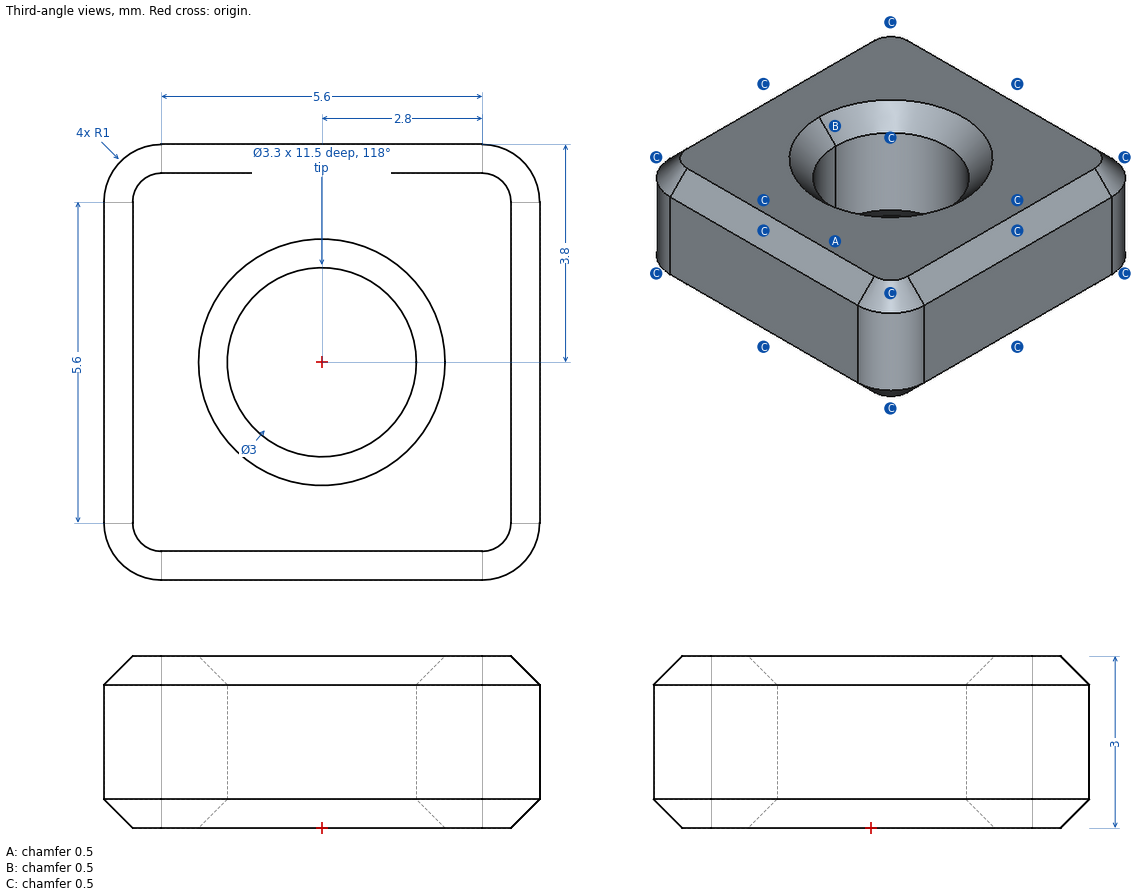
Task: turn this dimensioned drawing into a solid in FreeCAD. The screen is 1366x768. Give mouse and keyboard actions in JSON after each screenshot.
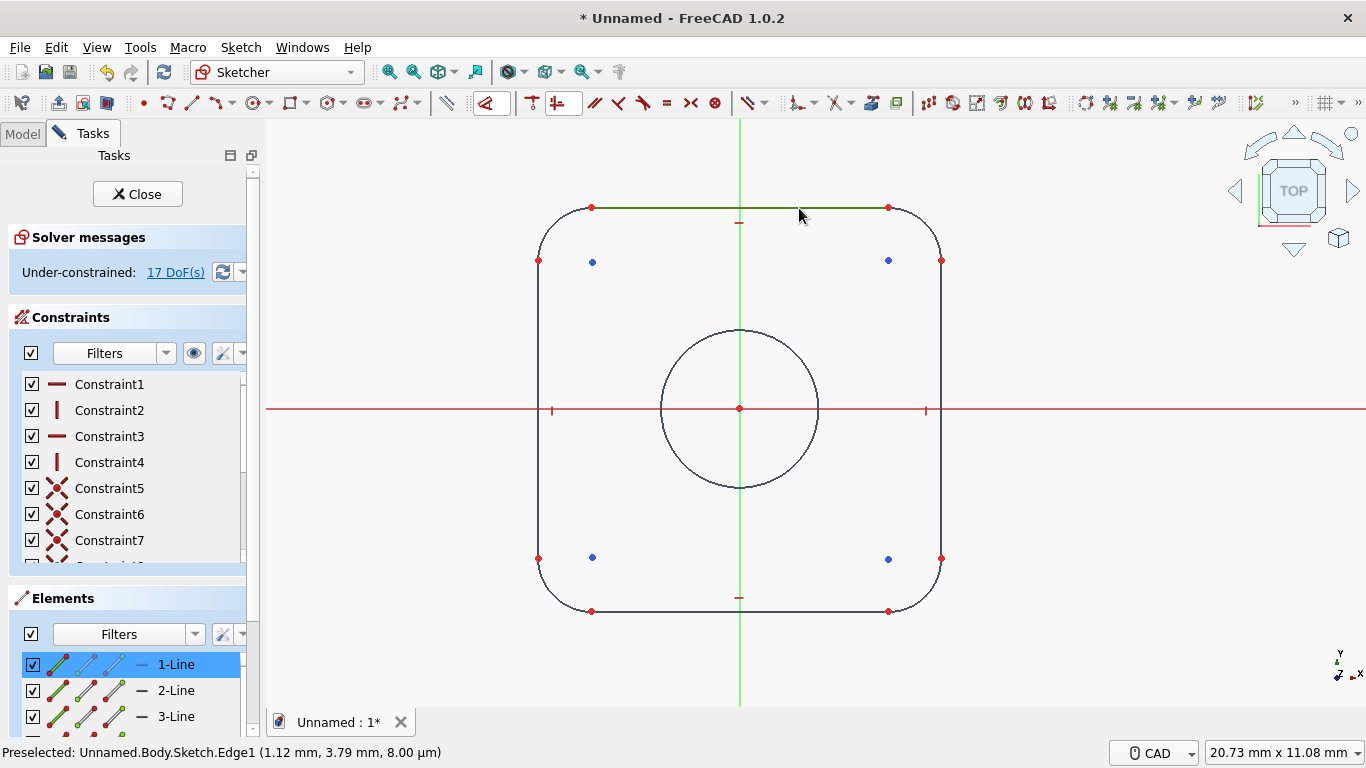
{"action": "left_click", "coordinate": [567, 214]}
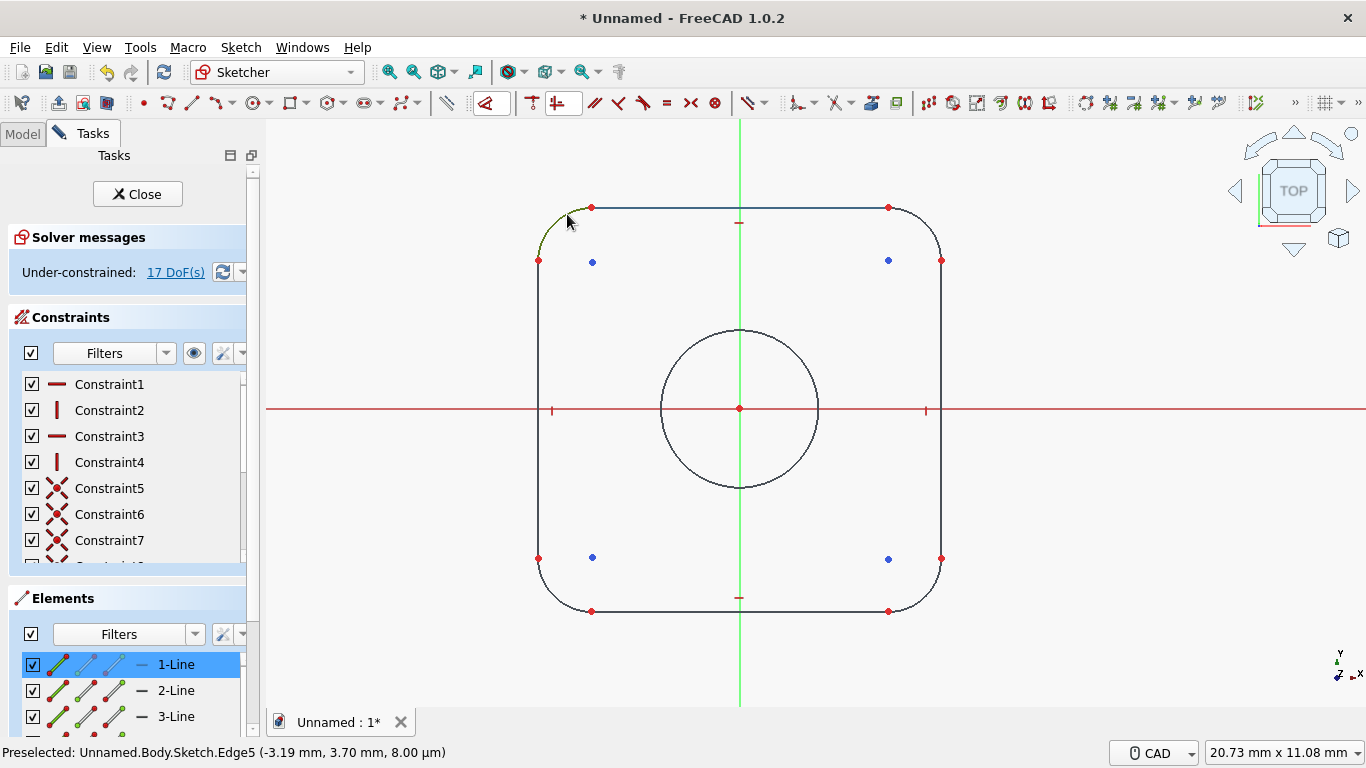
{"action": "key", "text": "t"}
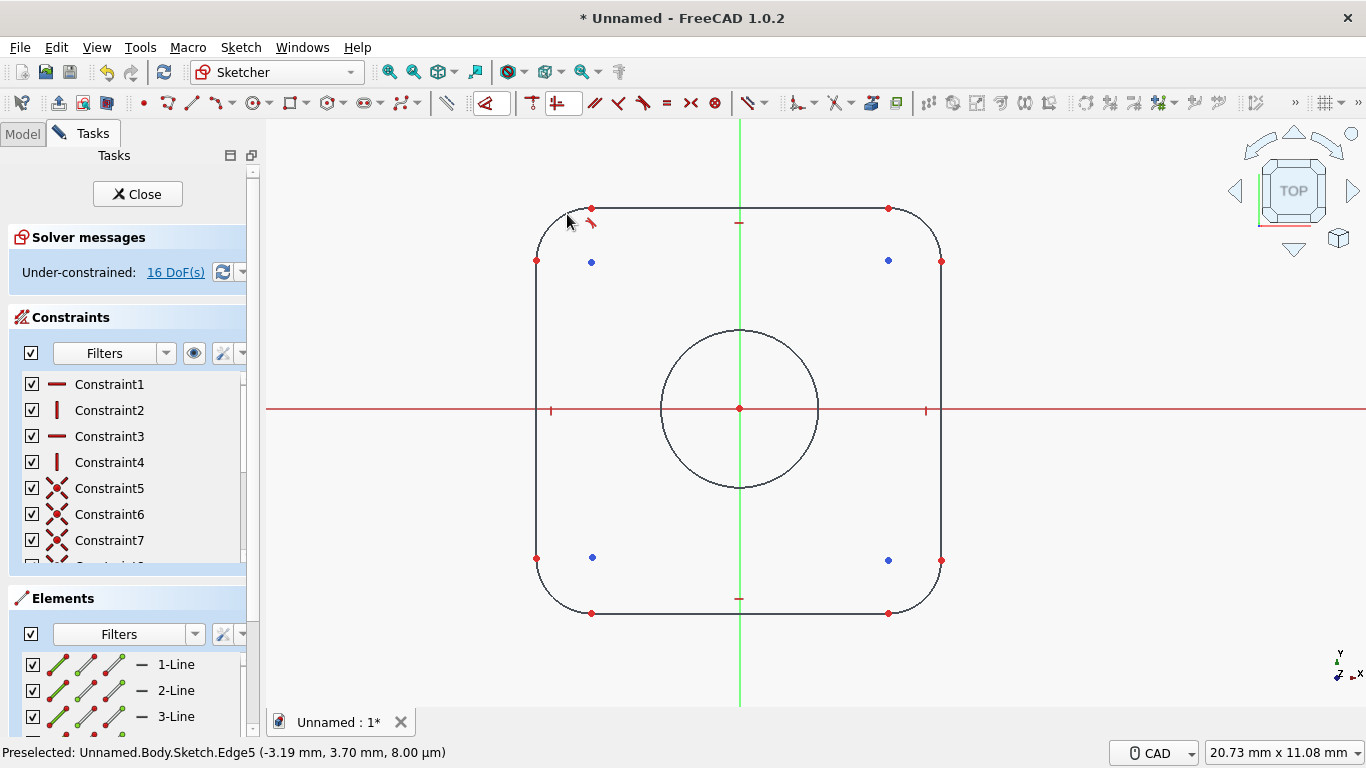
{"action": "left_click", "coordinate": [799, 208]}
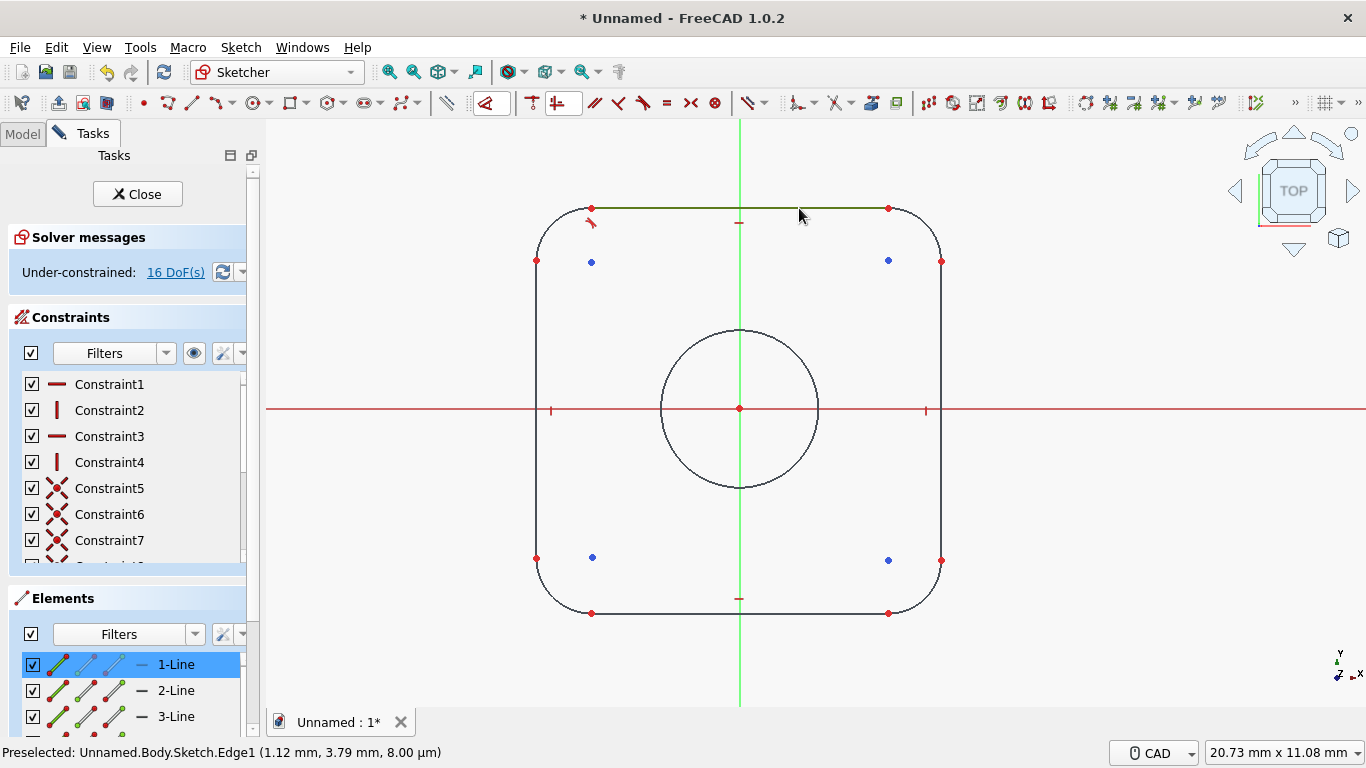
{"action": "left_click", "coordinate": [935, 237]}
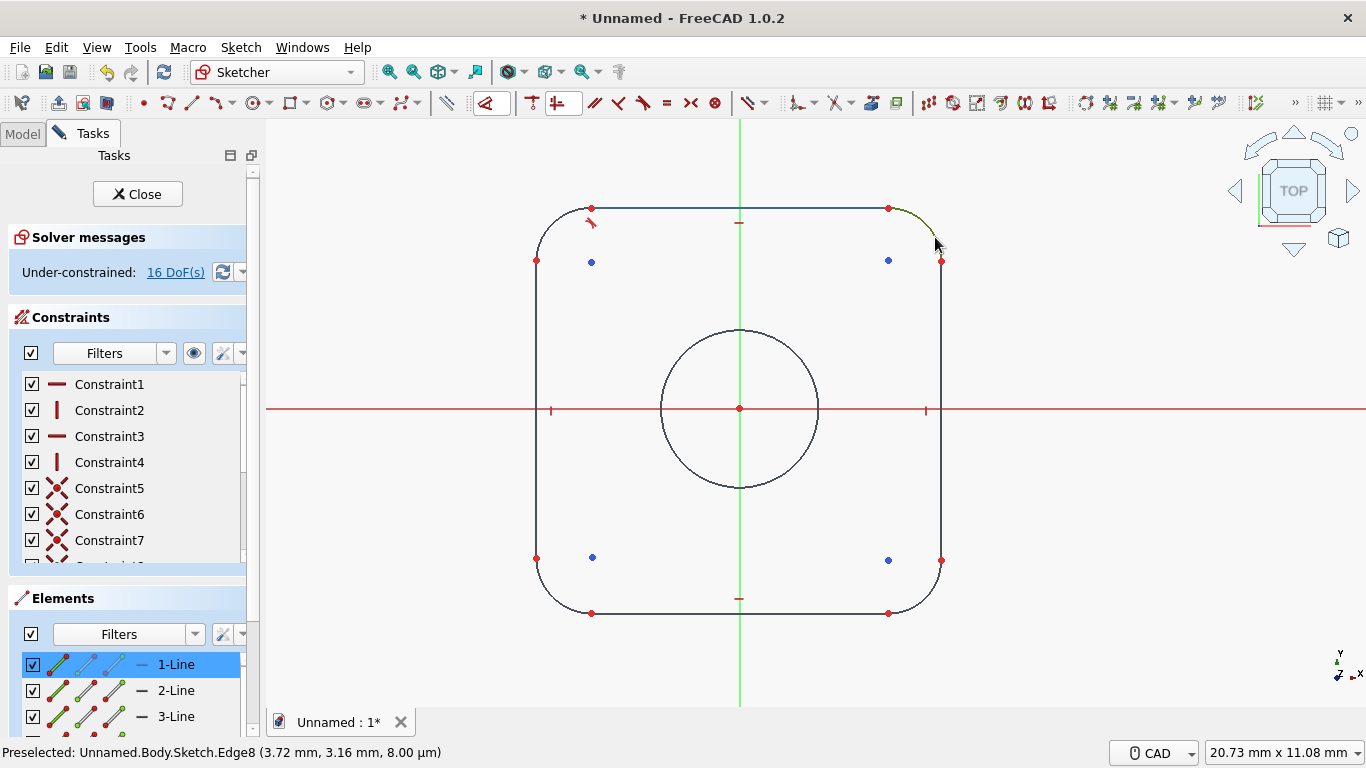
{"action": "left_click", "coordinate": [644, 104]}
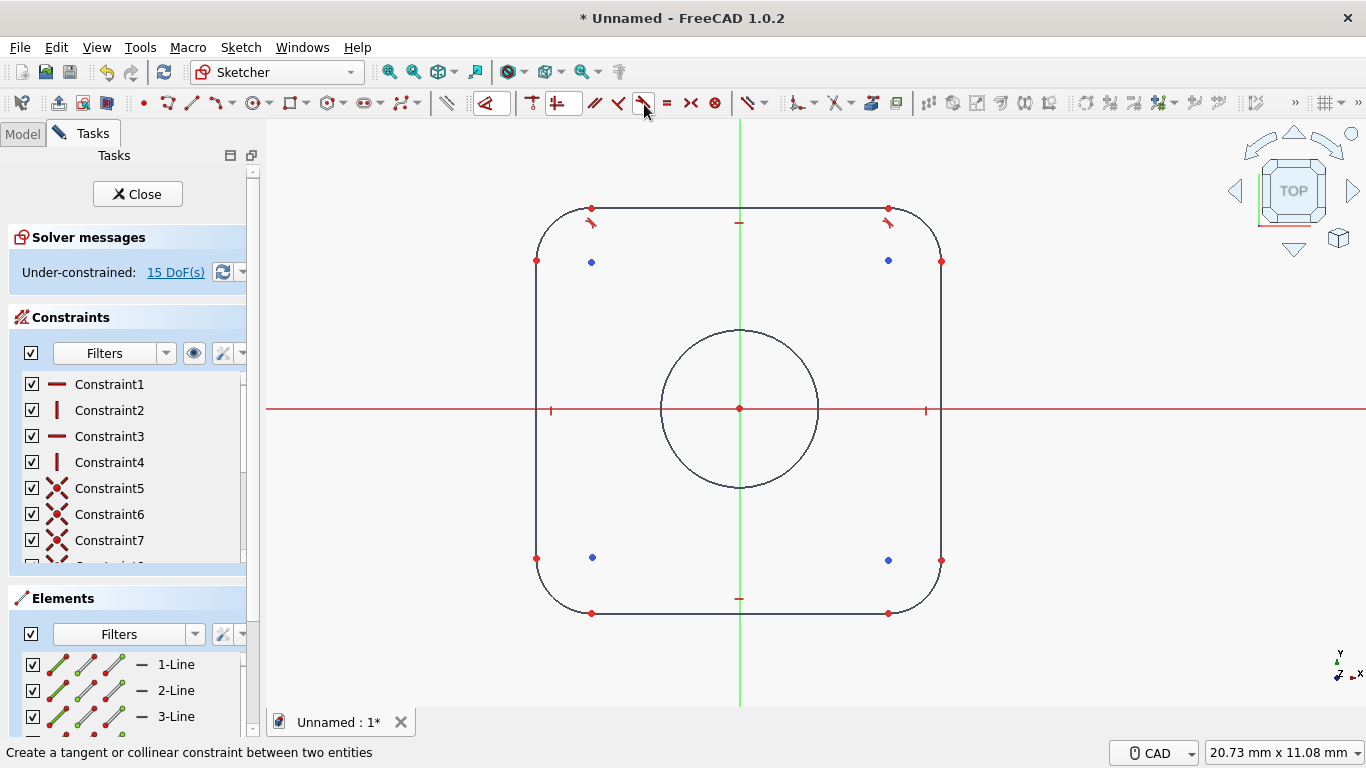
{"action": "left_click", "coordinate": [536, 350]}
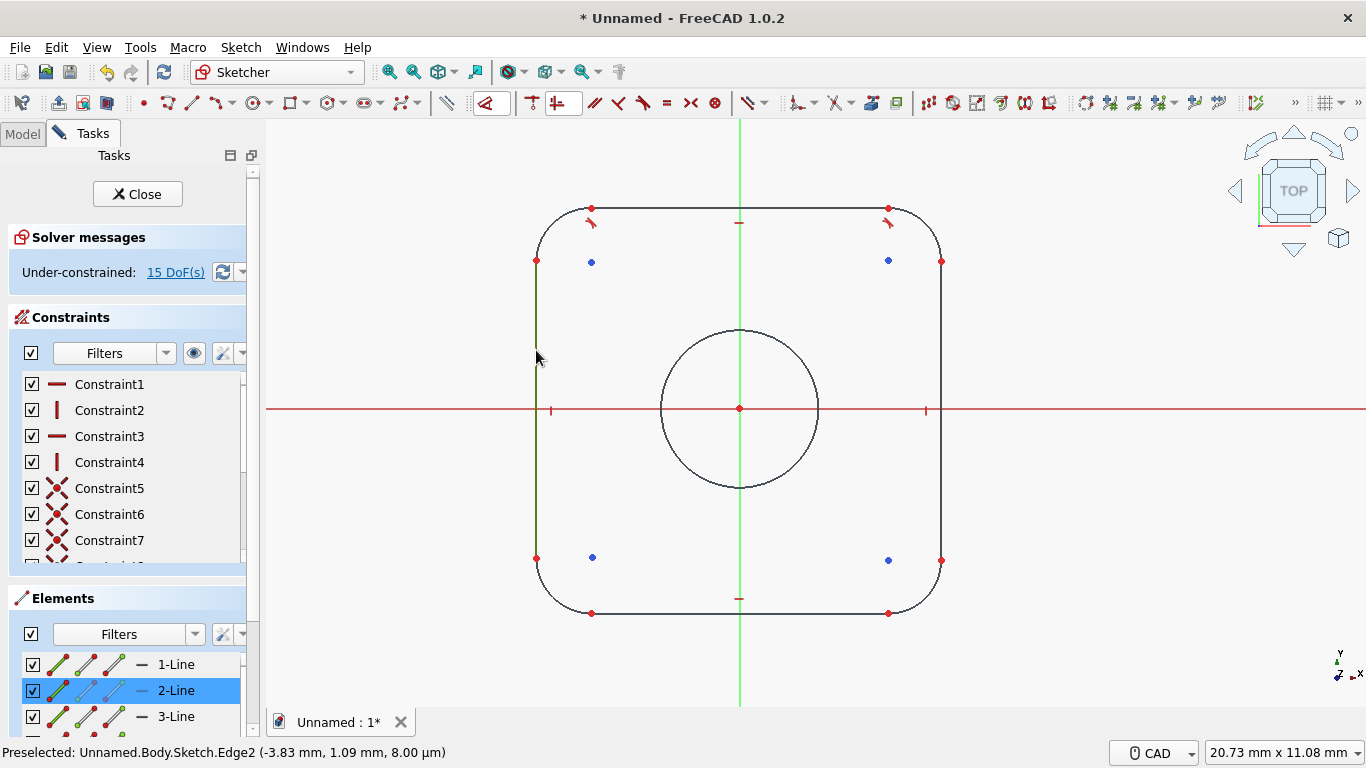
{"action": "left_click", "coordinate": [567, 214]}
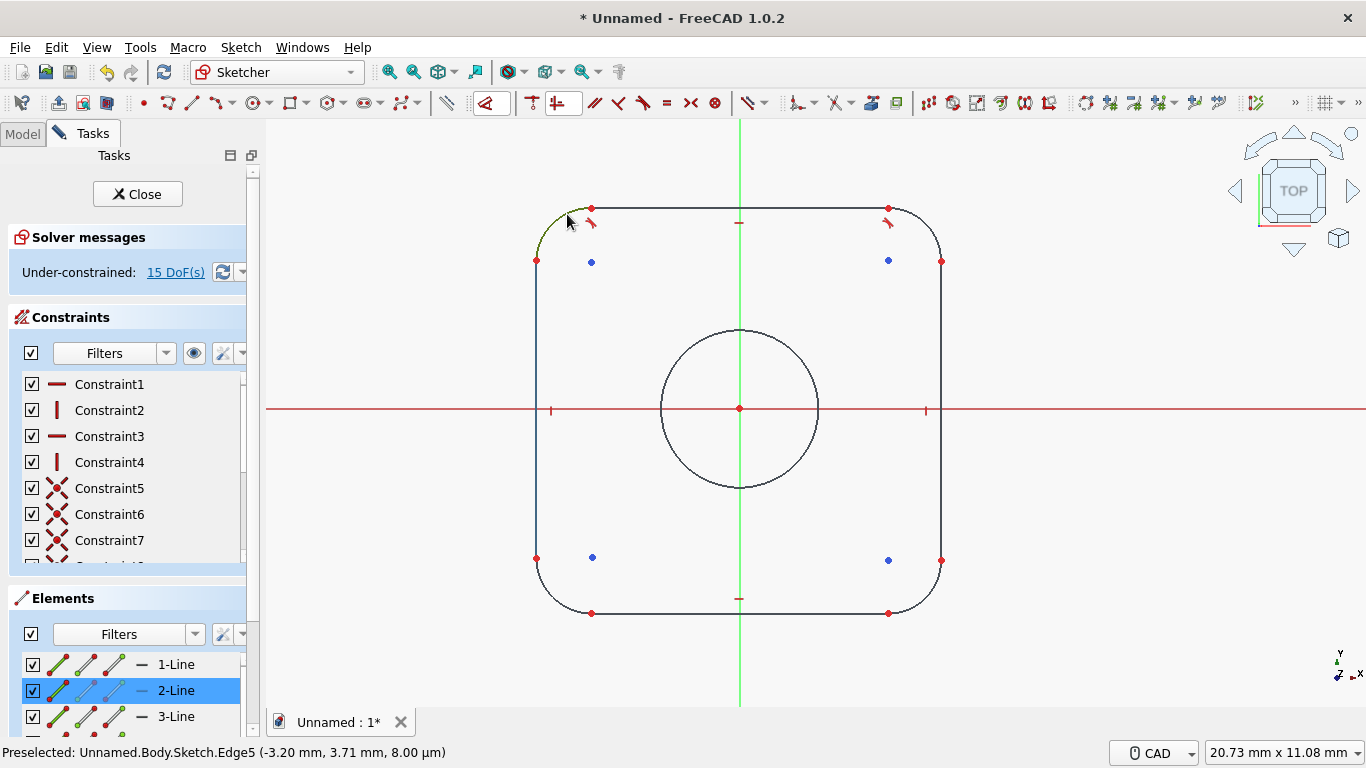
{"action": "key", "text": "t"}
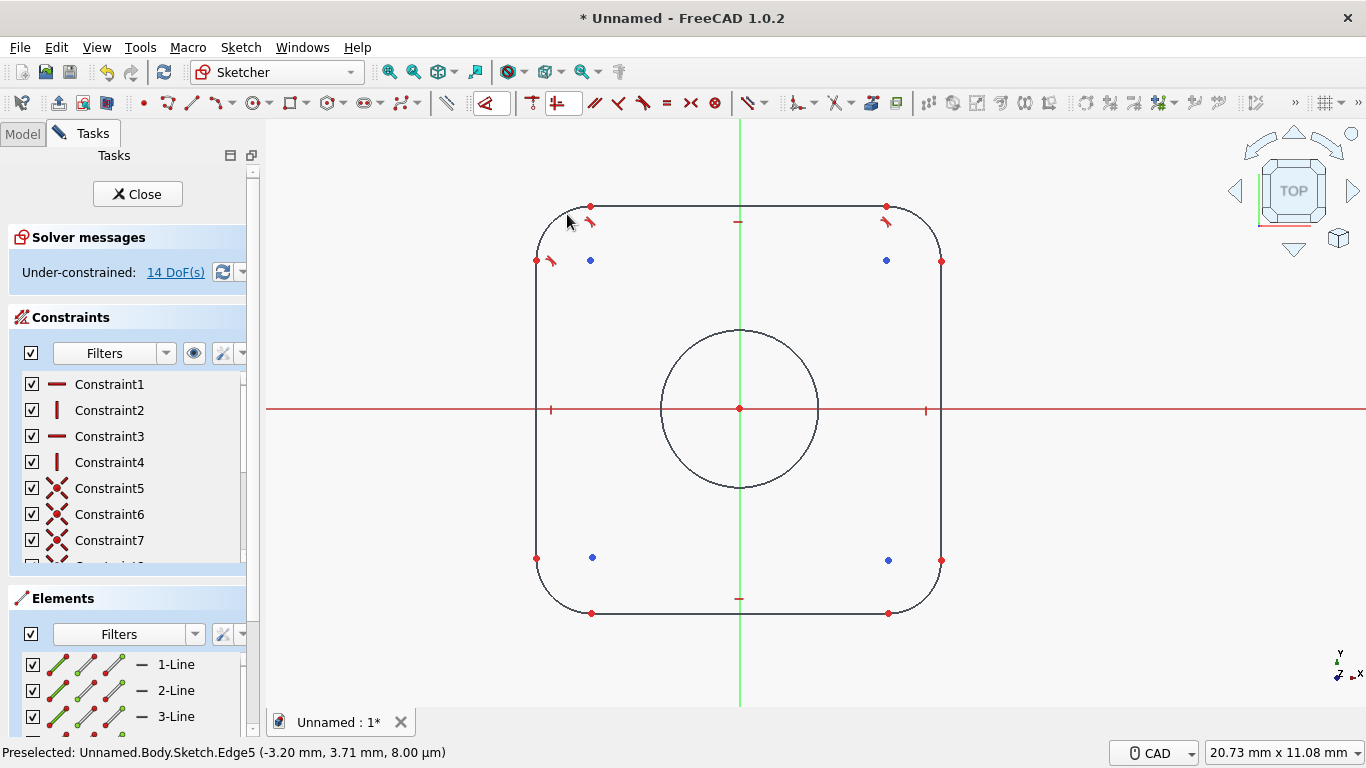
{"action": "left_click", "coordinate": [536, 350]}